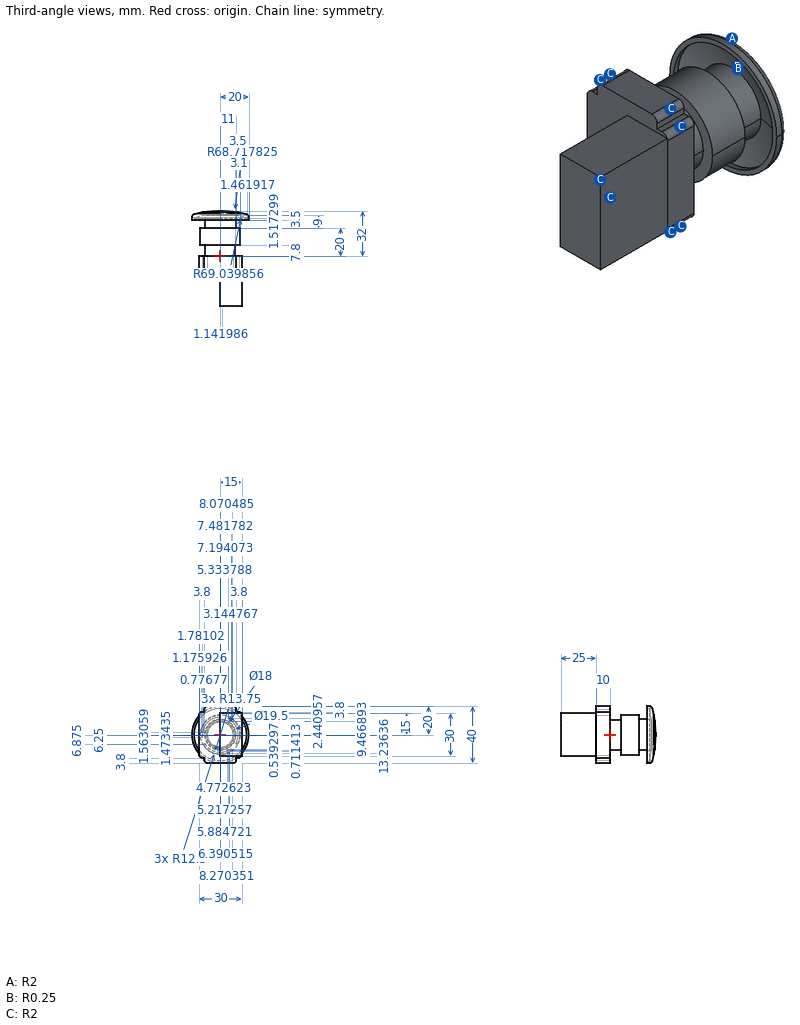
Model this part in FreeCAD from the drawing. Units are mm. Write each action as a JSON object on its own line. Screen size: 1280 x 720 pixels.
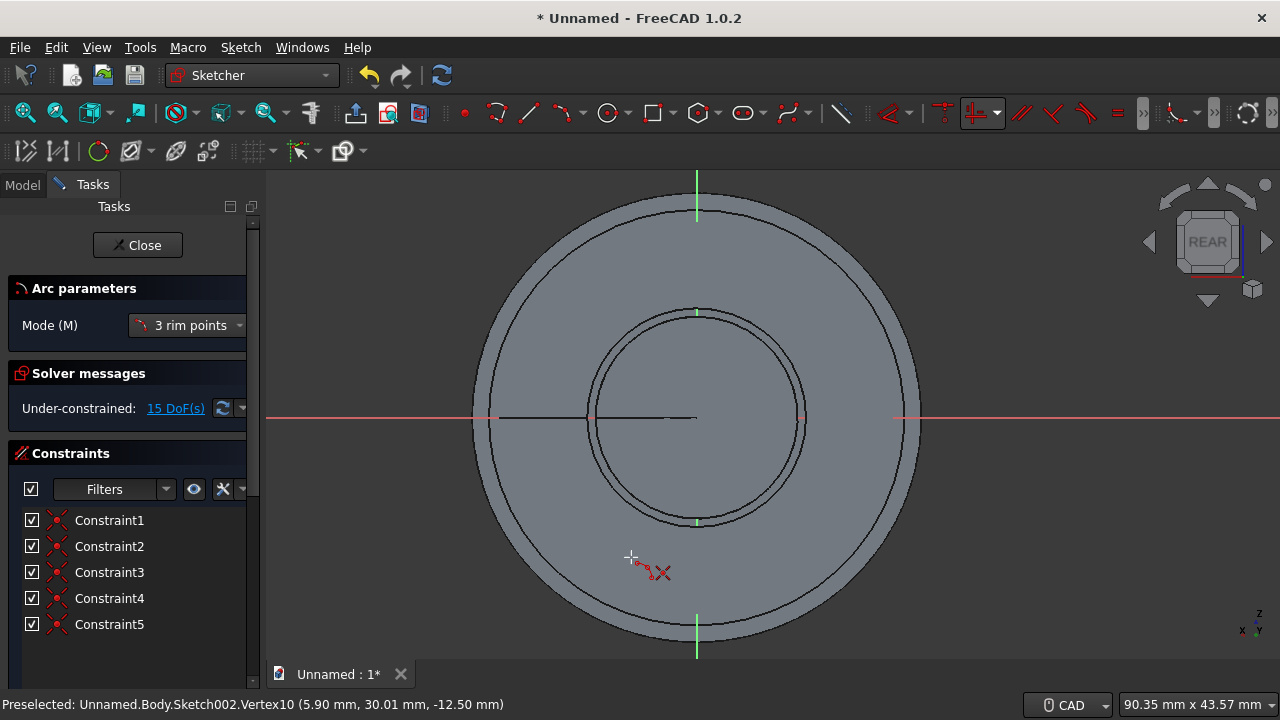
{"action": "scroll", "coordinate": [830, 495], "scroll_direction": "up", "scroll_amount": 5}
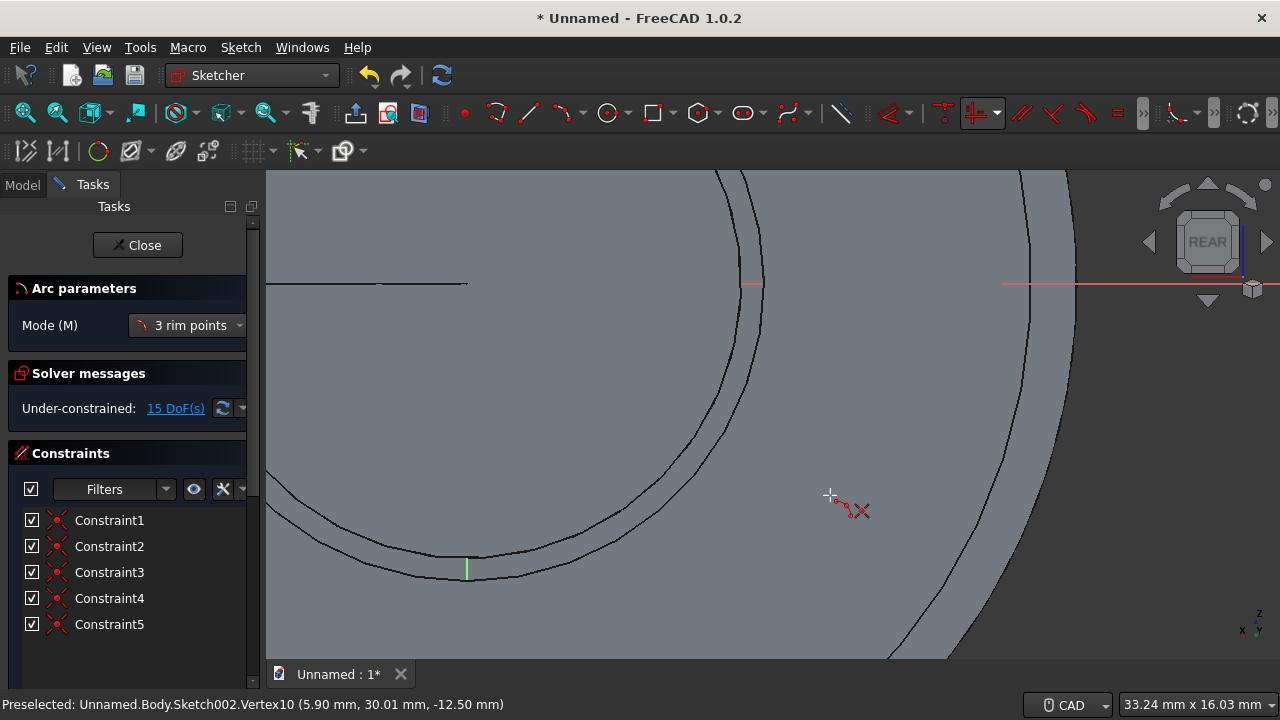
{"action": "left_click", "coordinate": [829, 497]}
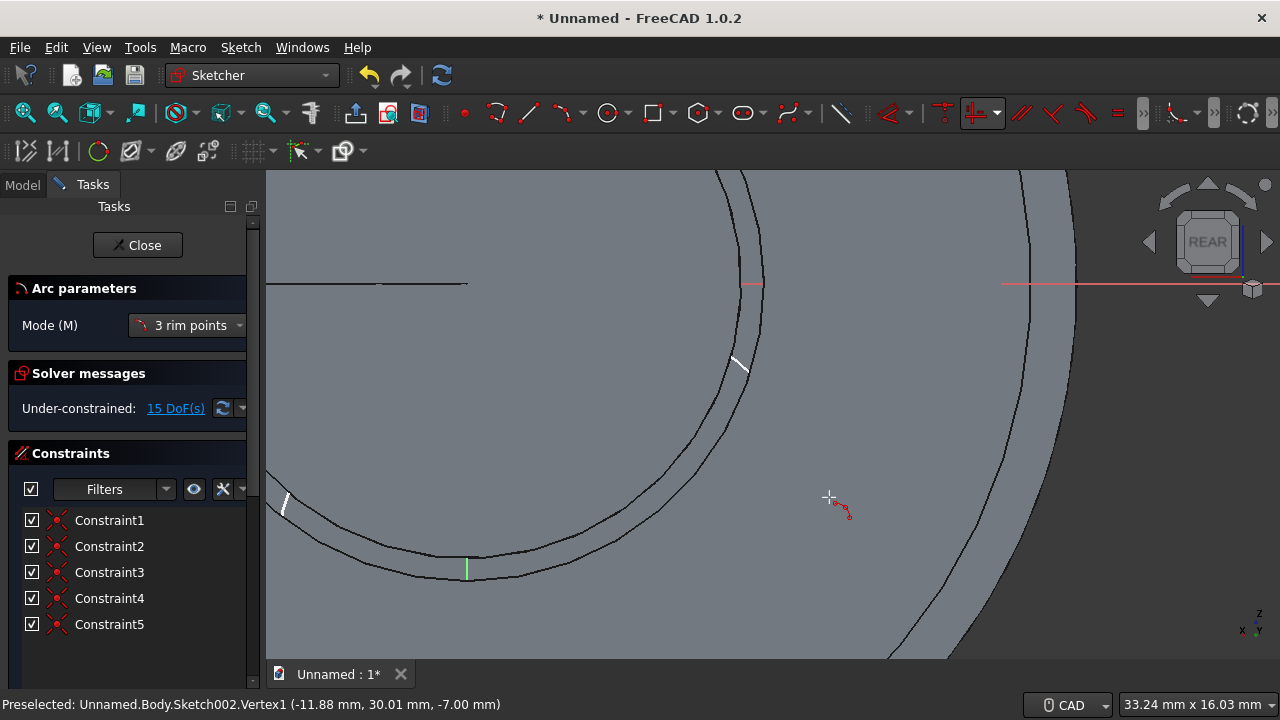
{"action": "scroll", "coordinate": [831, 495], "scroll_direction": "down", "scroll_amount": 5}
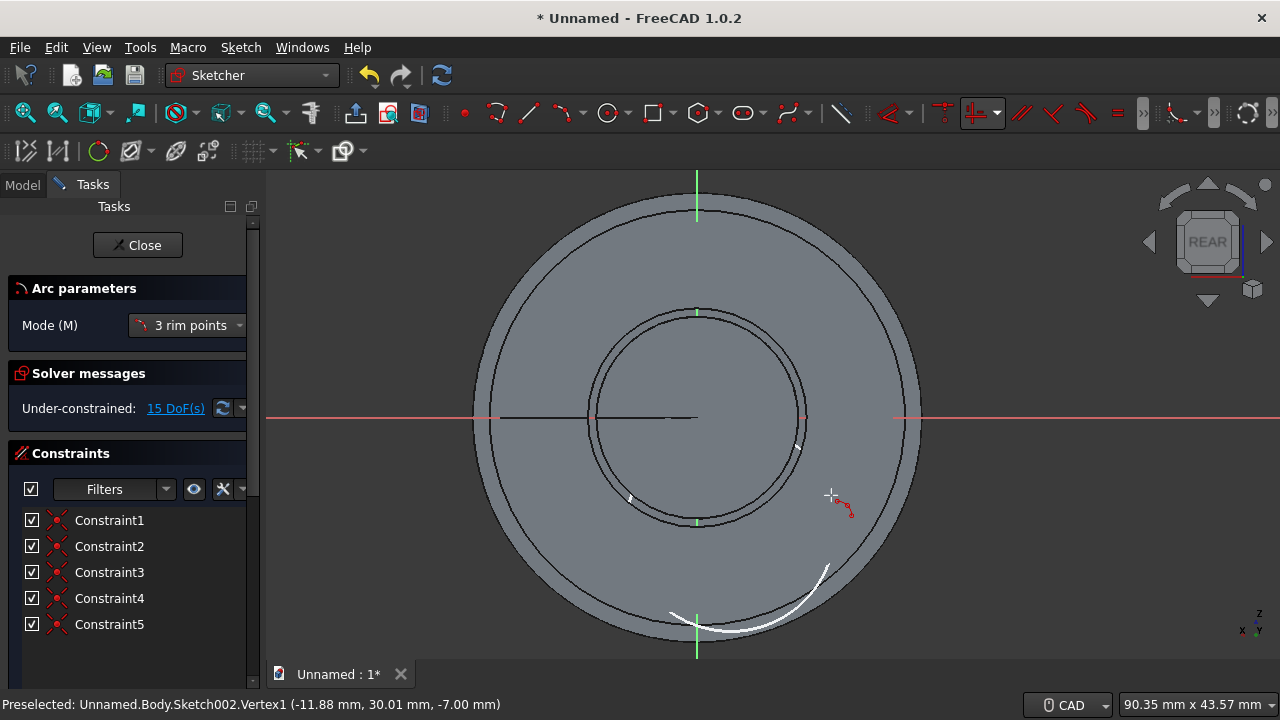
{"action": "left_click", "coordinate": [743, 565]}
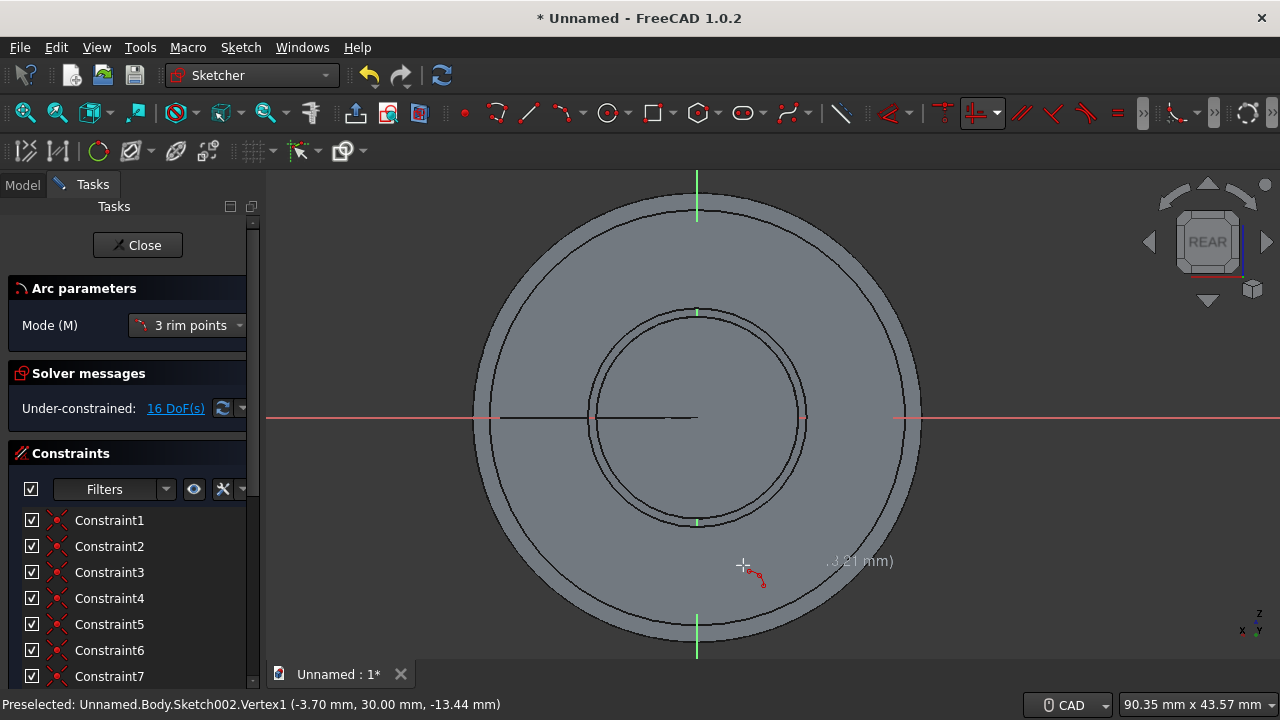
{"action": "left_click", "coordinate": [530, 114]}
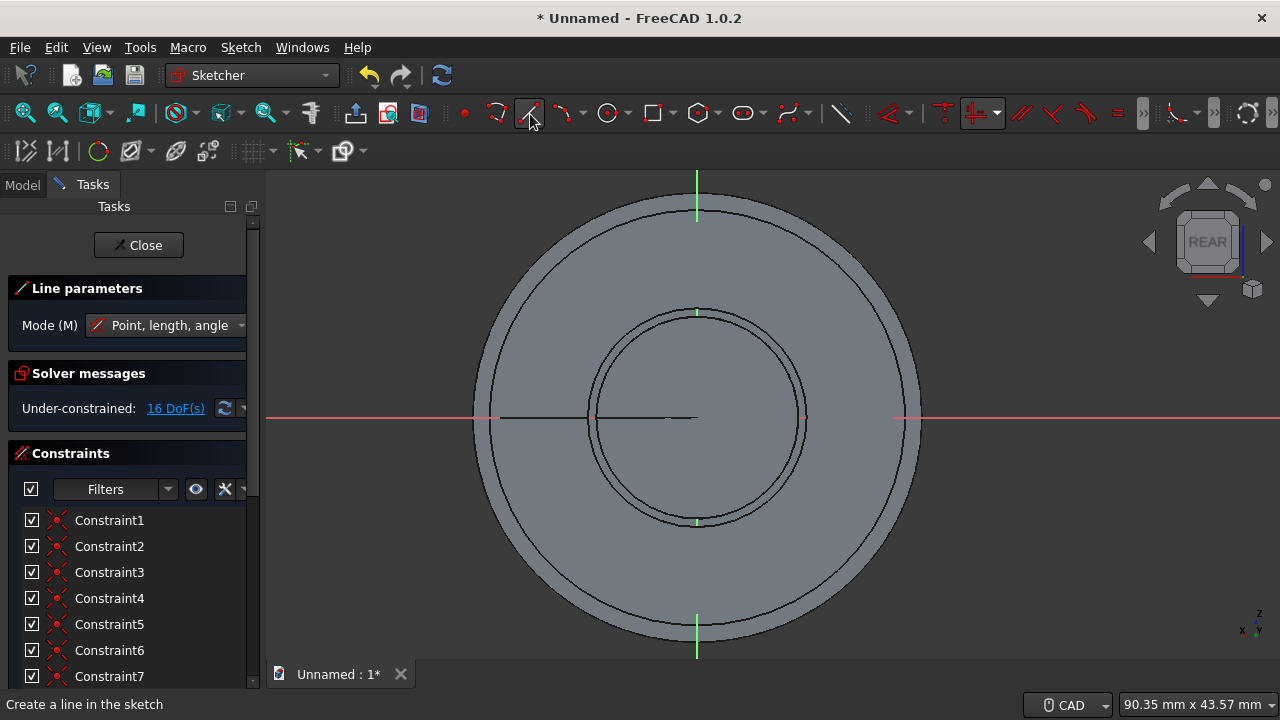
{"action": "left_click", "coordinate": [697, 263]}
{"action": "left_click", "coordinate": [706, 277]}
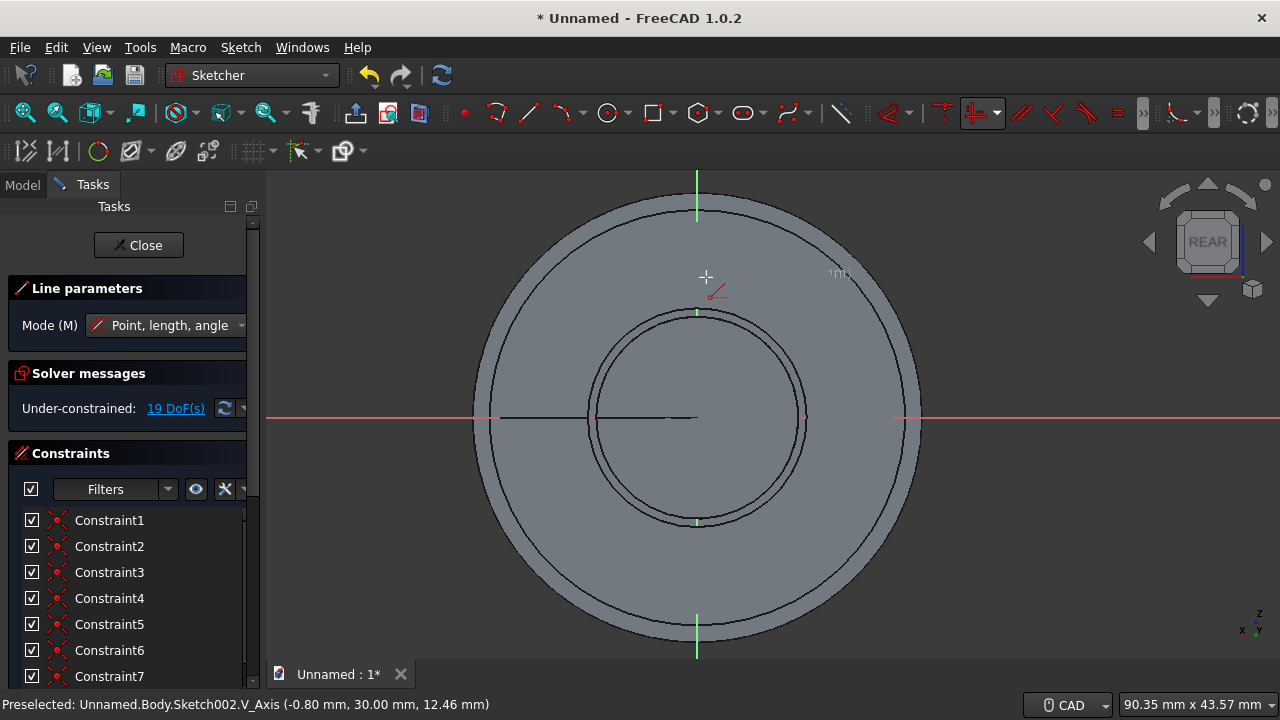
{"action": "left_click", "coordinate": [498, 114]}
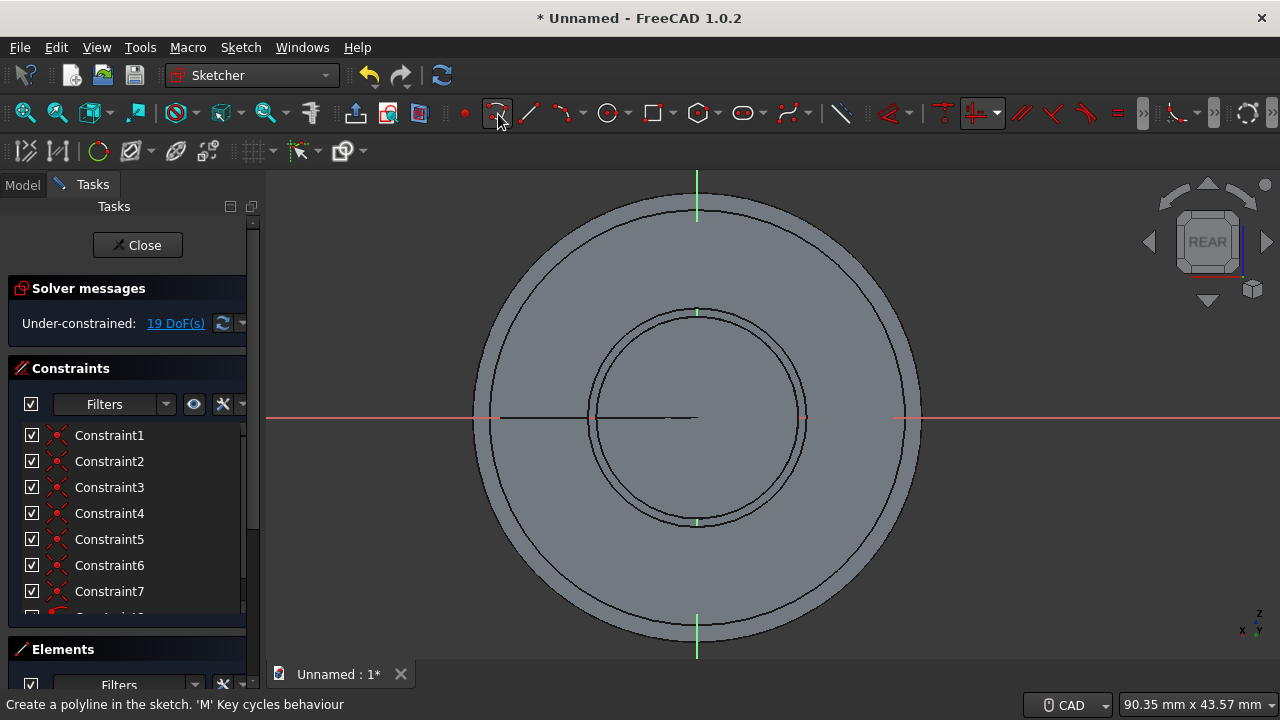
{"action": "left_click", "coordinate": [836, 400]}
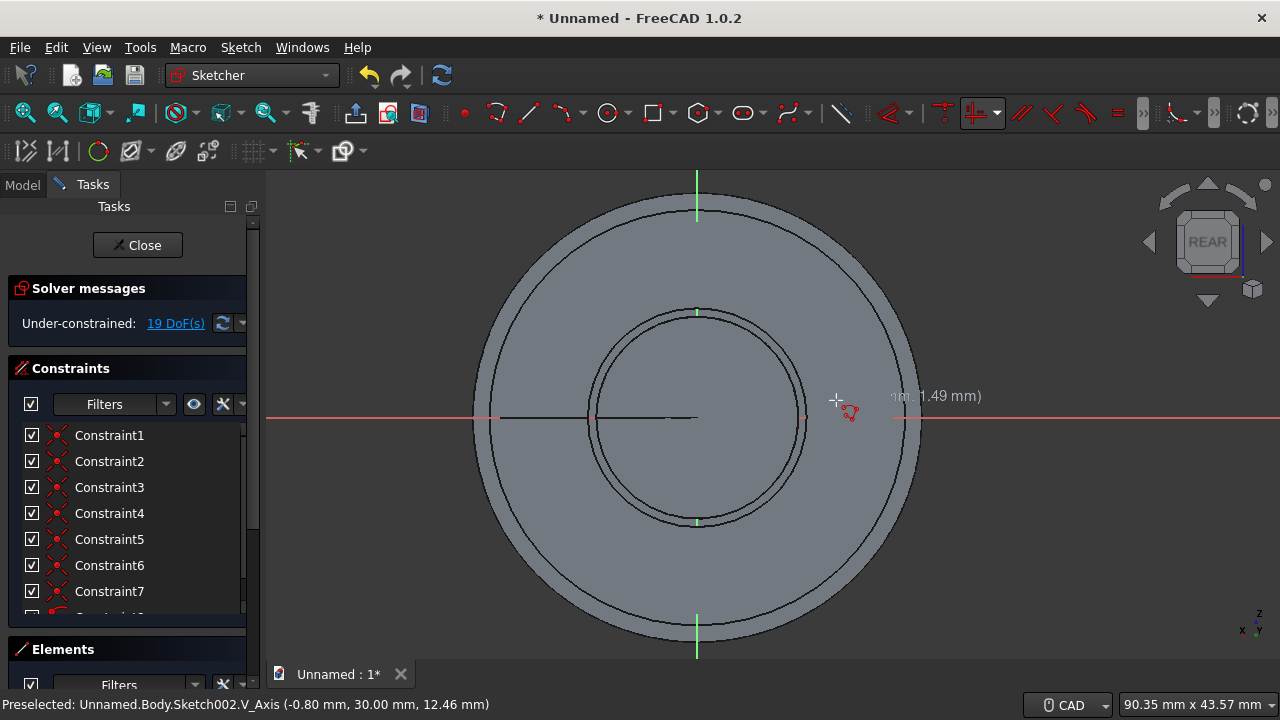
{"action": "scroll", "coordinate": [828, 400], "scroll_direction": "up", "scroll_amount": 3}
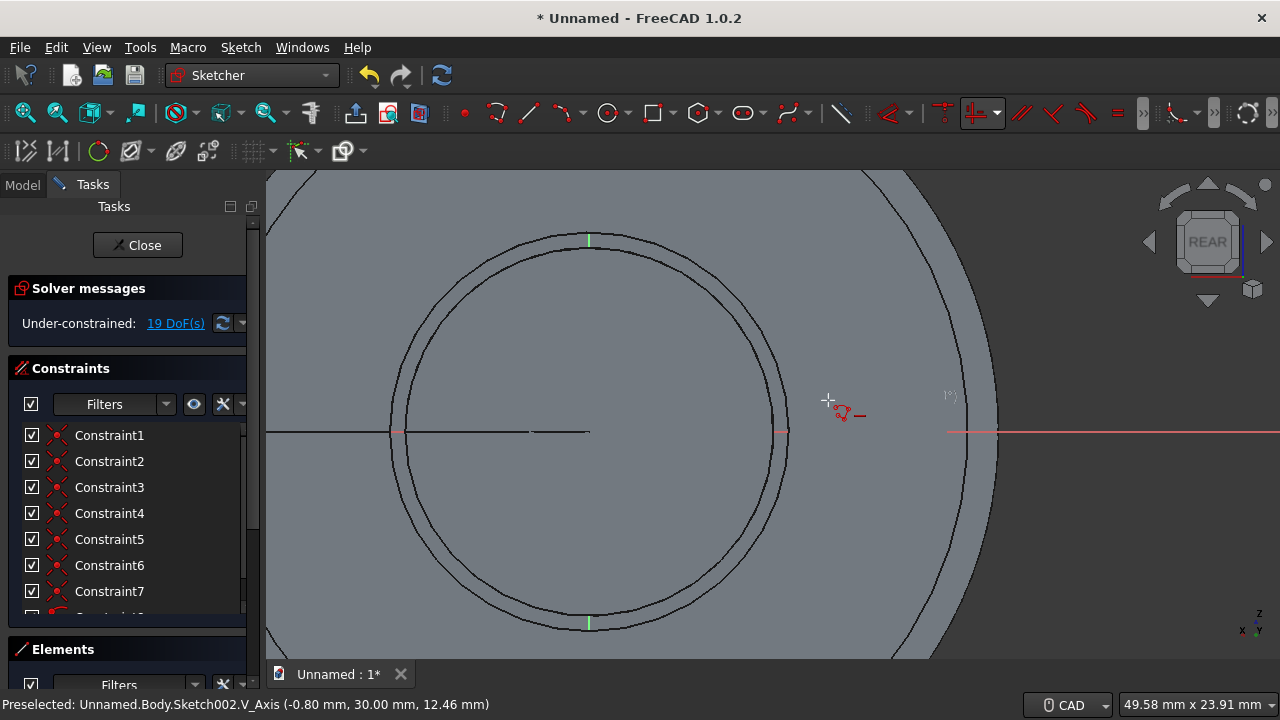
{"action": "left_click", "coordinate": [827, 400]}
{"action": "left_click", "coordinate": [856, 462]}
{"action": "left_click", "coordinate": [893, 400]}
{"action": "left_click", "coordinate": [869, 400]}
{"action": "right_click", "coordinate": [869, 400]}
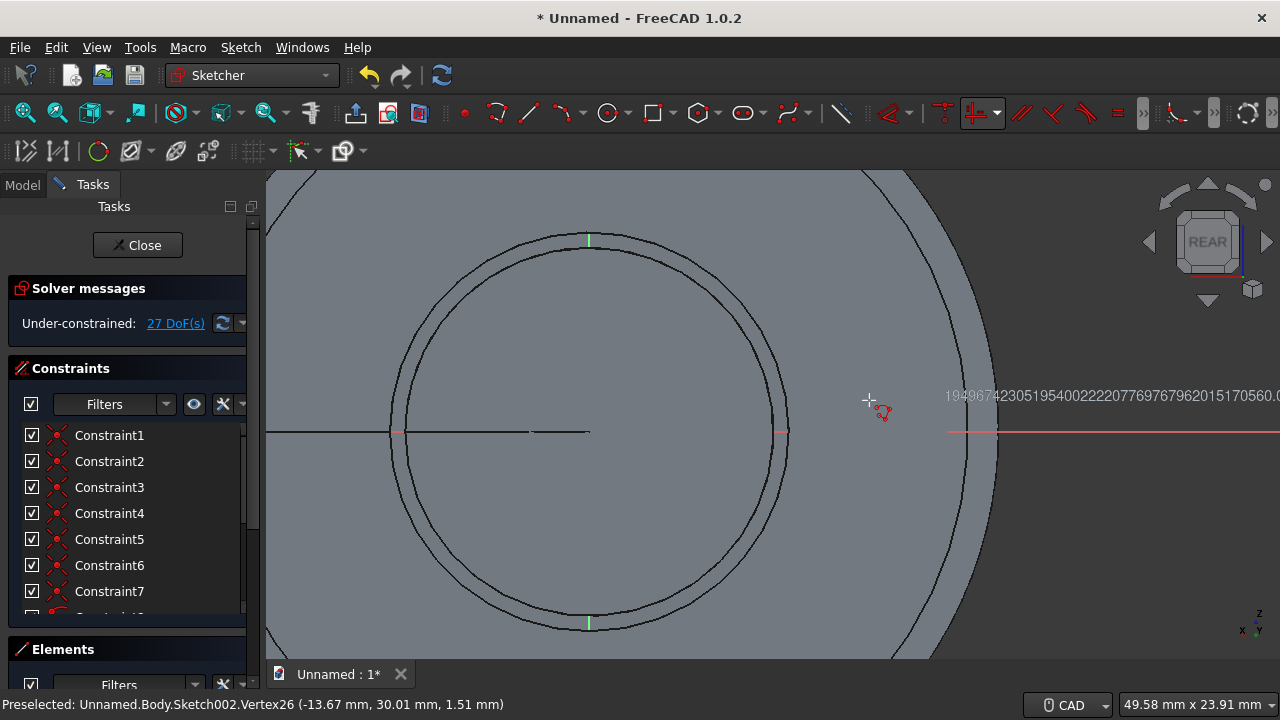
{"action": "left_click", "coordinate": [562, 114]}